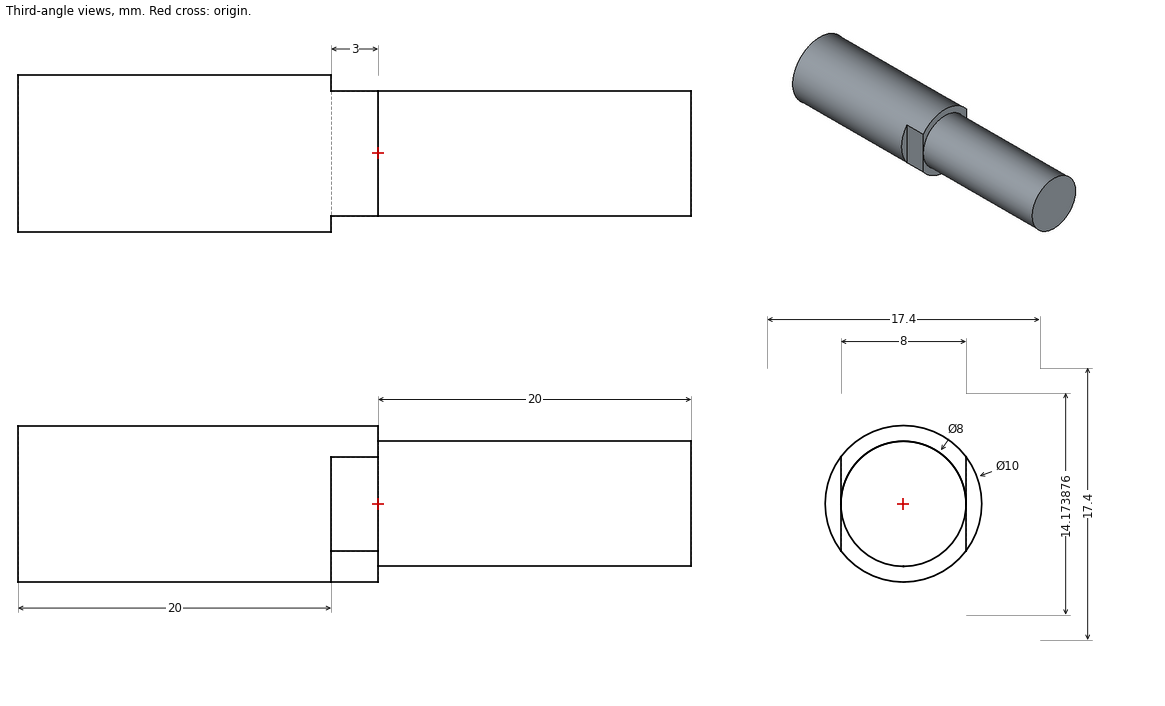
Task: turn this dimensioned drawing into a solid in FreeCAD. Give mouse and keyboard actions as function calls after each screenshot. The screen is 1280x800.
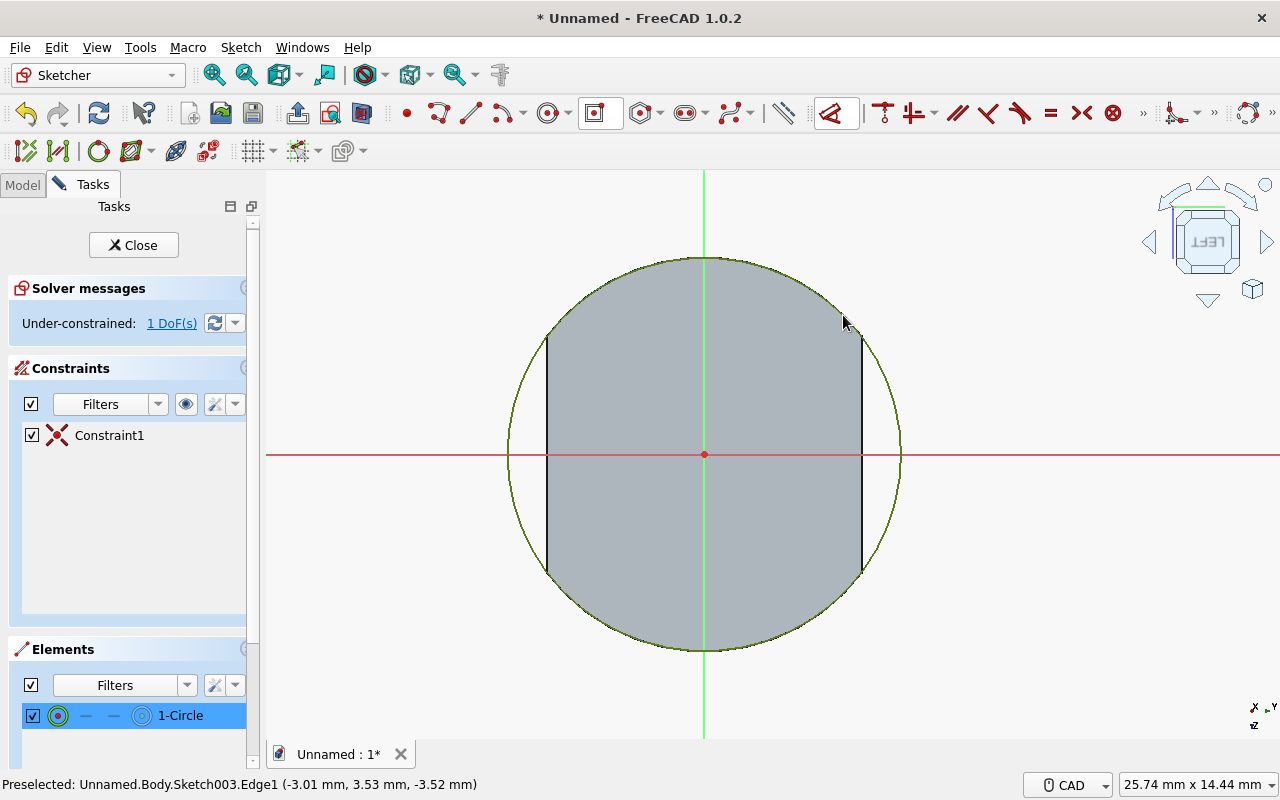
click(854, 114)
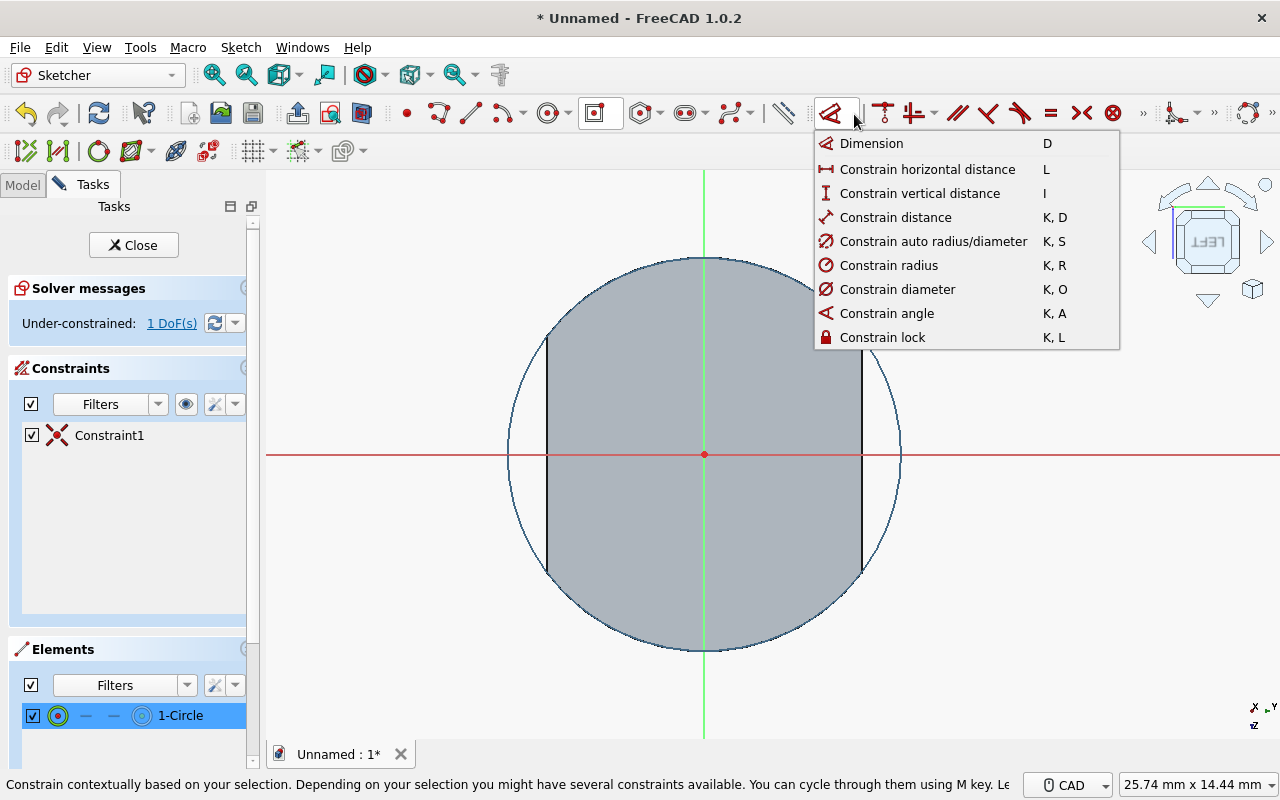
click(967, 289)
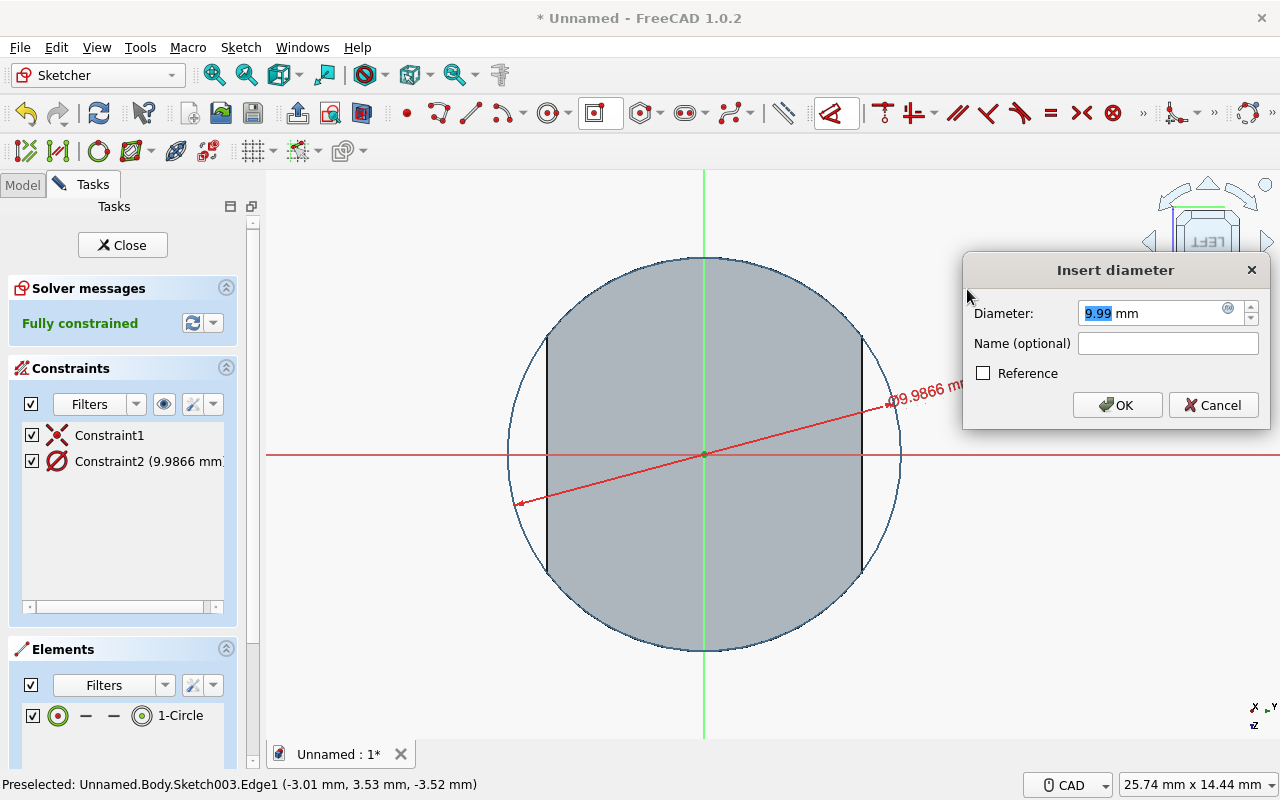
text(10)
key(Return)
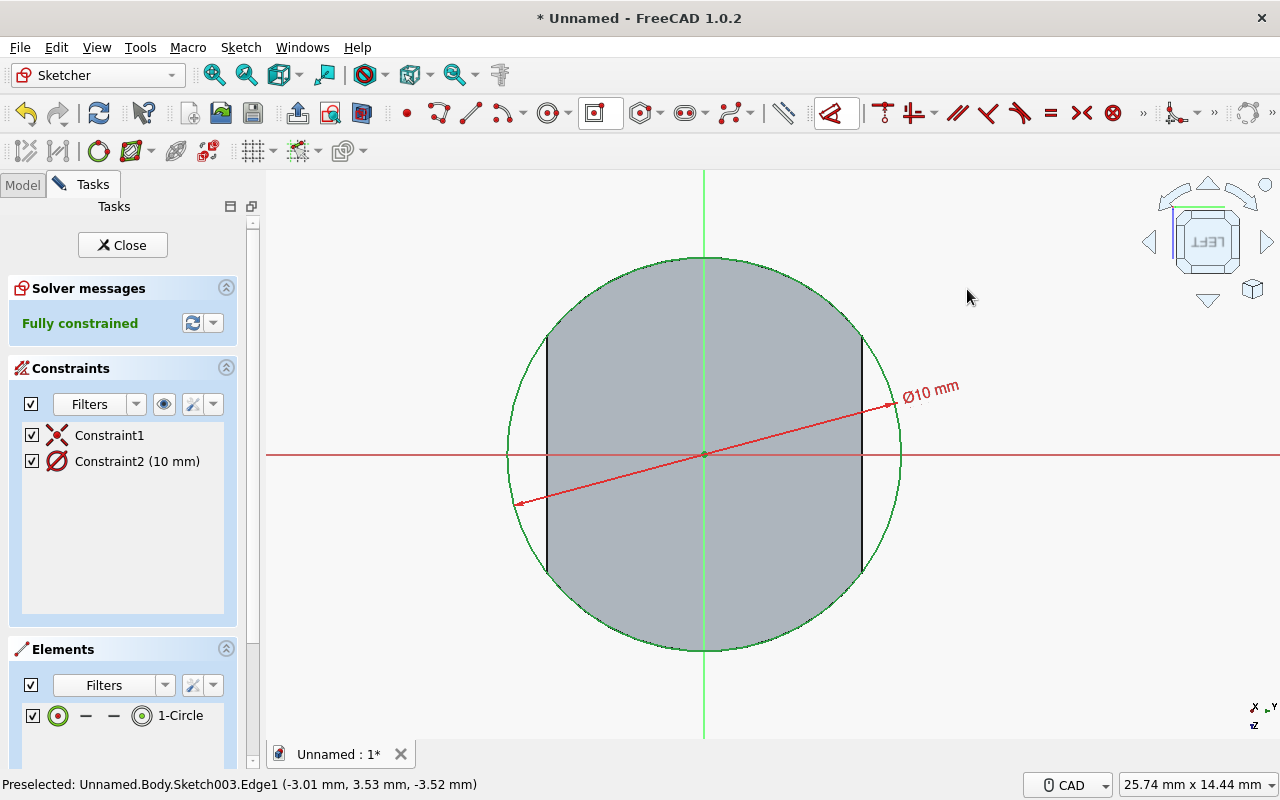
click(123, 245)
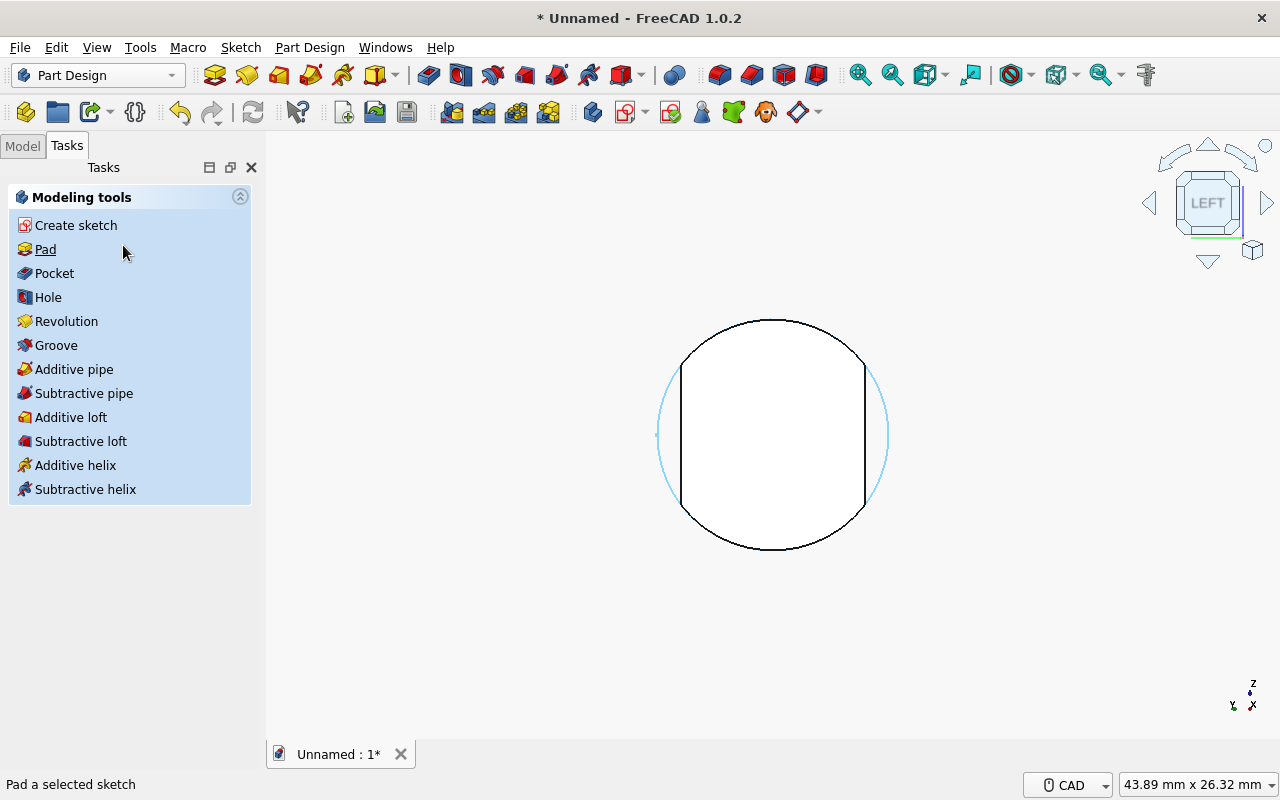
click(216, 76)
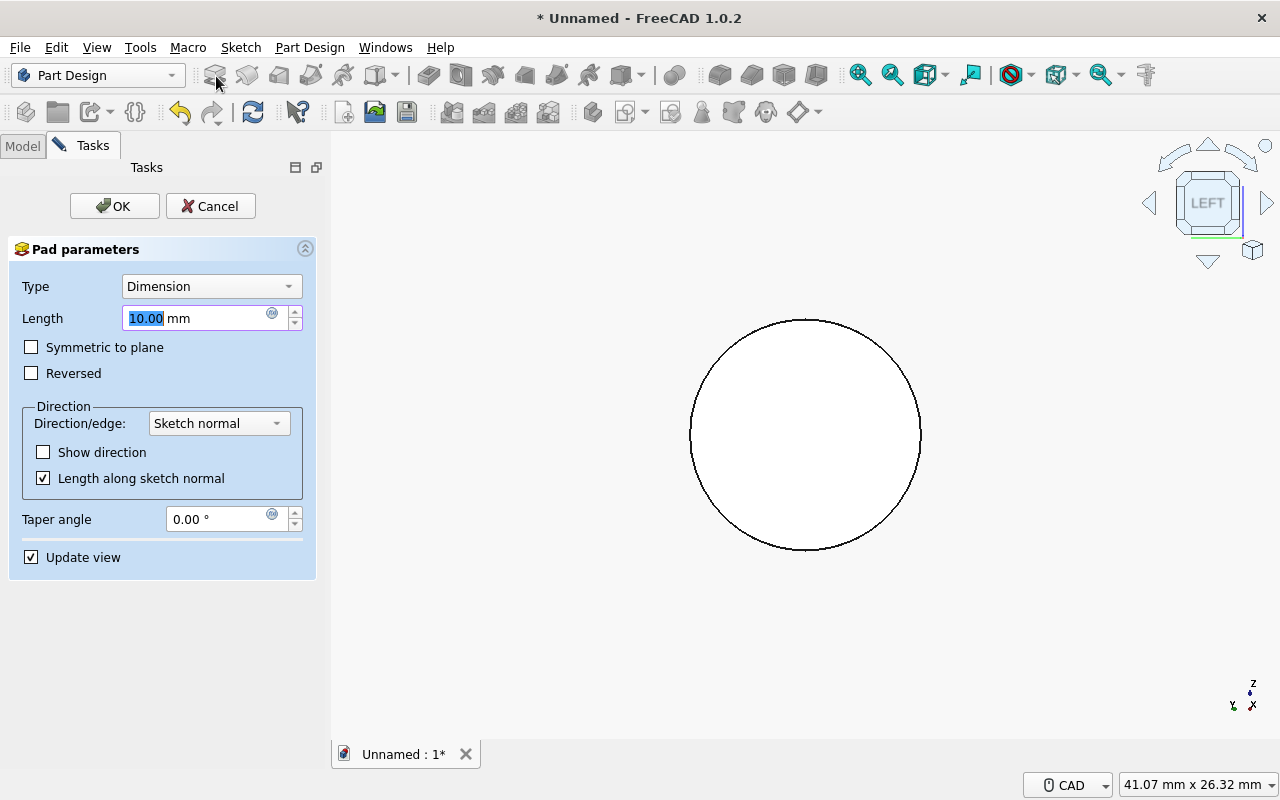
text(20)
key(Tab)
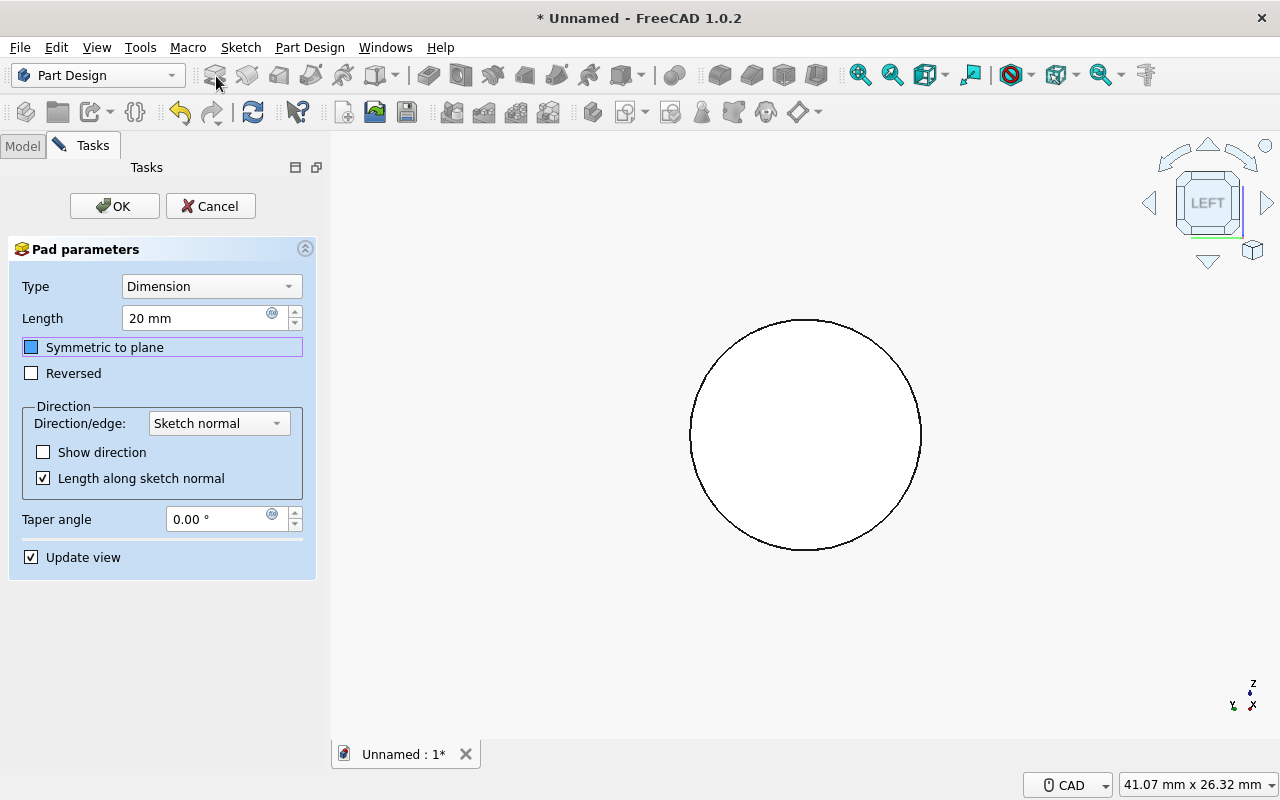
click(115, 206)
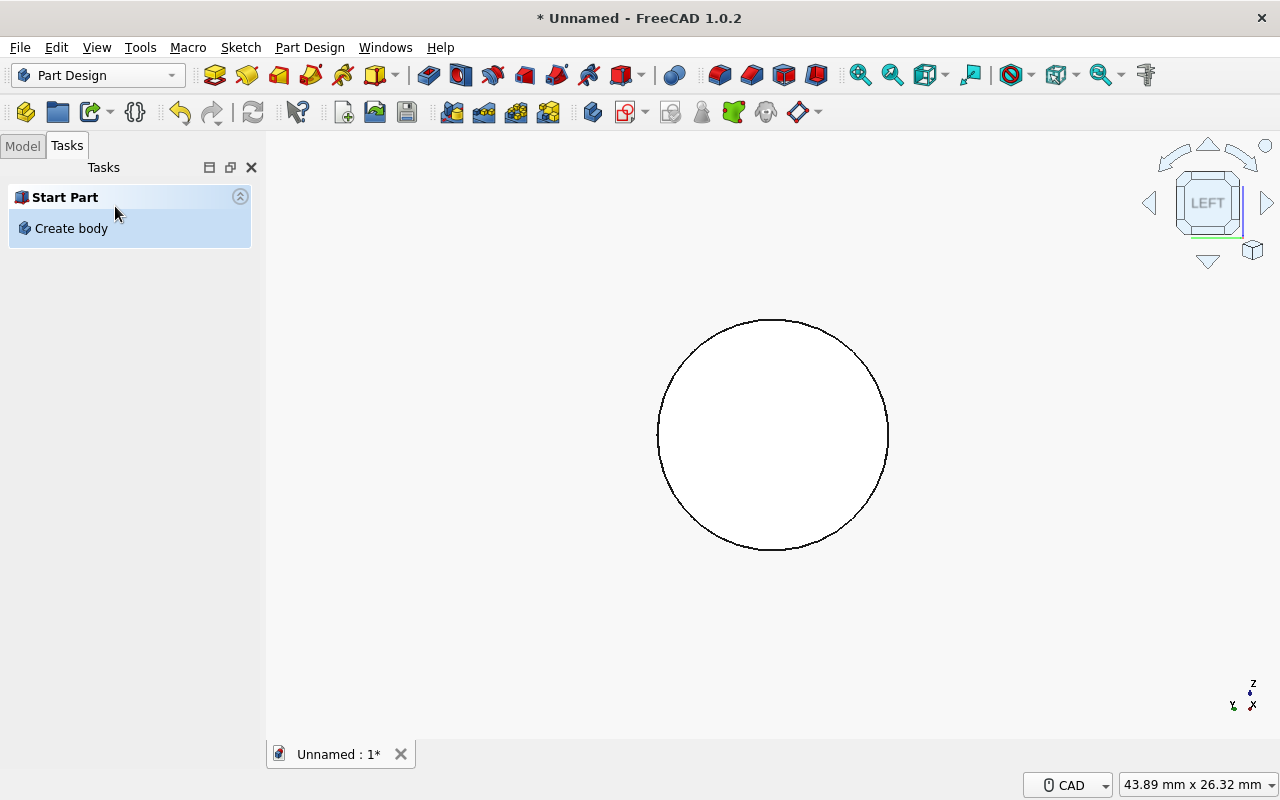
key(0)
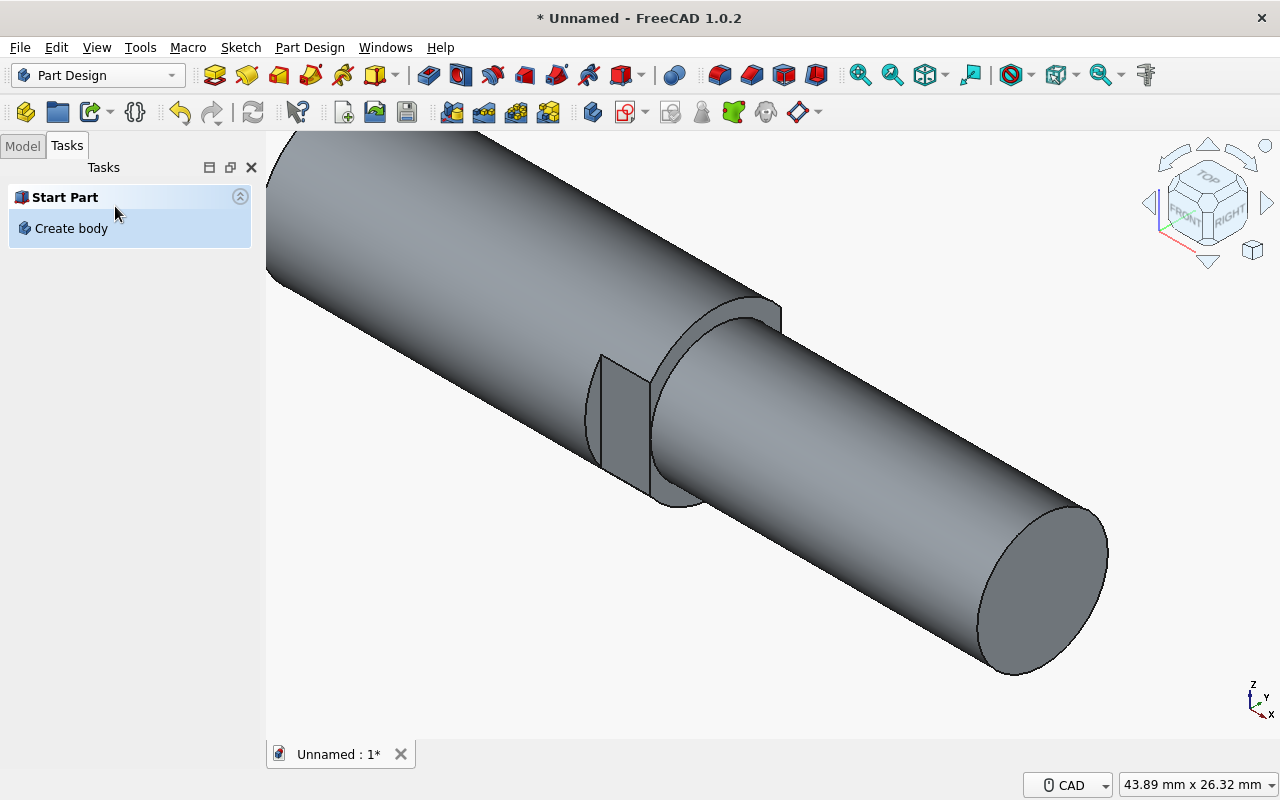
click(862, 76)